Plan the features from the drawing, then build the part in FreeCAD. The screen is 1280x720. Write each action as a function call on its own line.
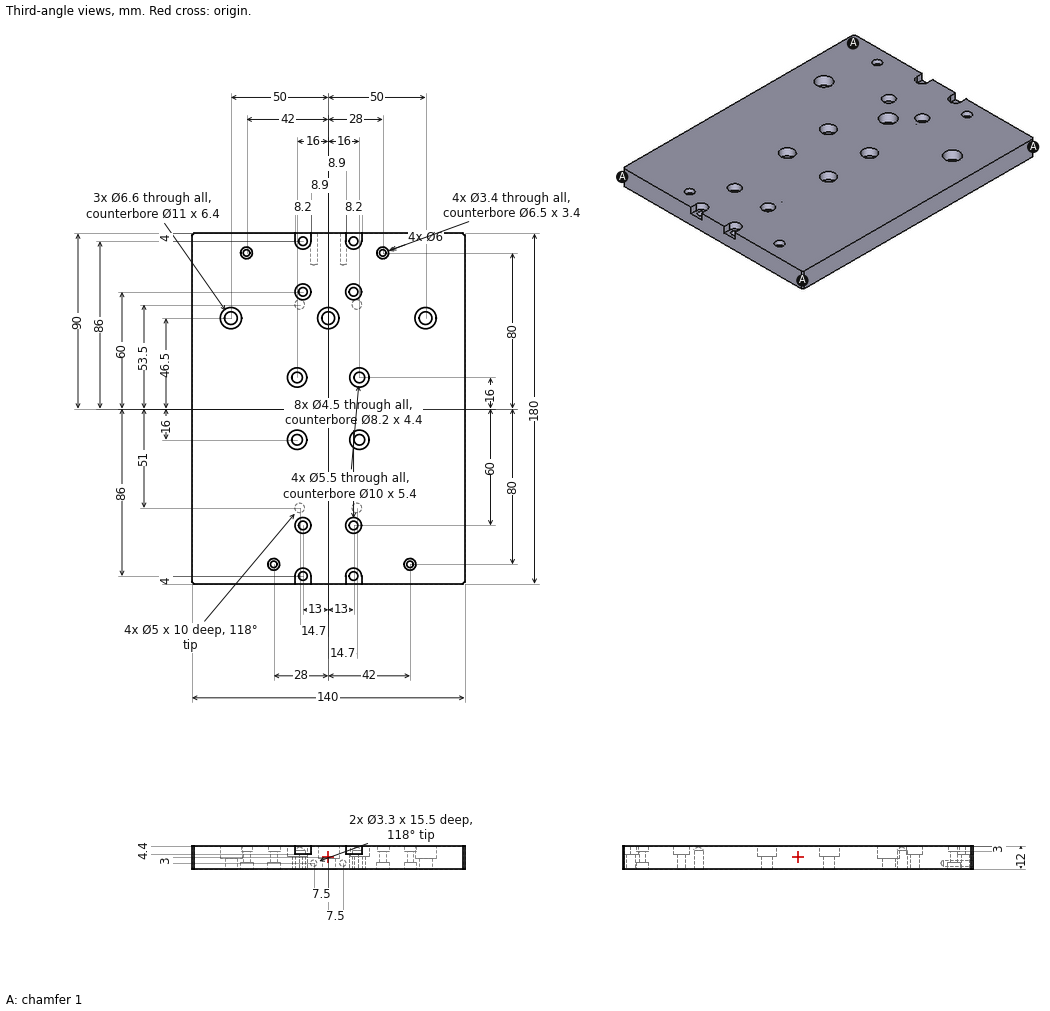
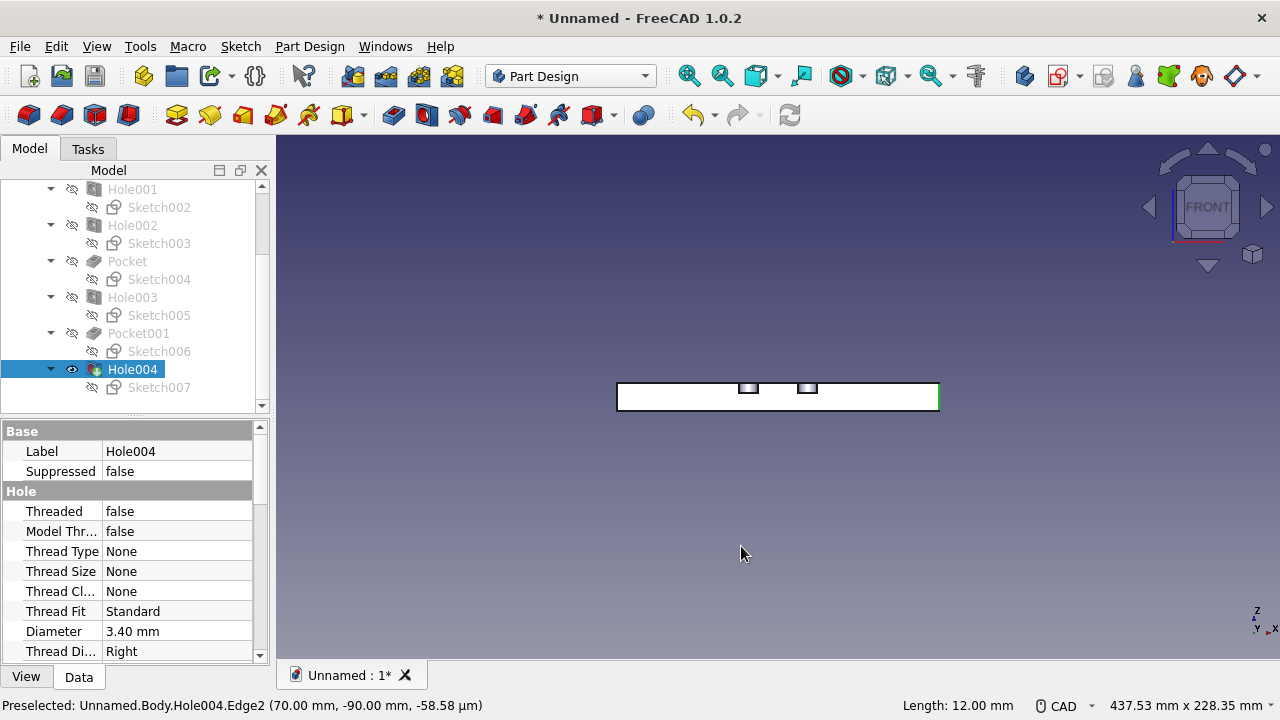
click(690, 76)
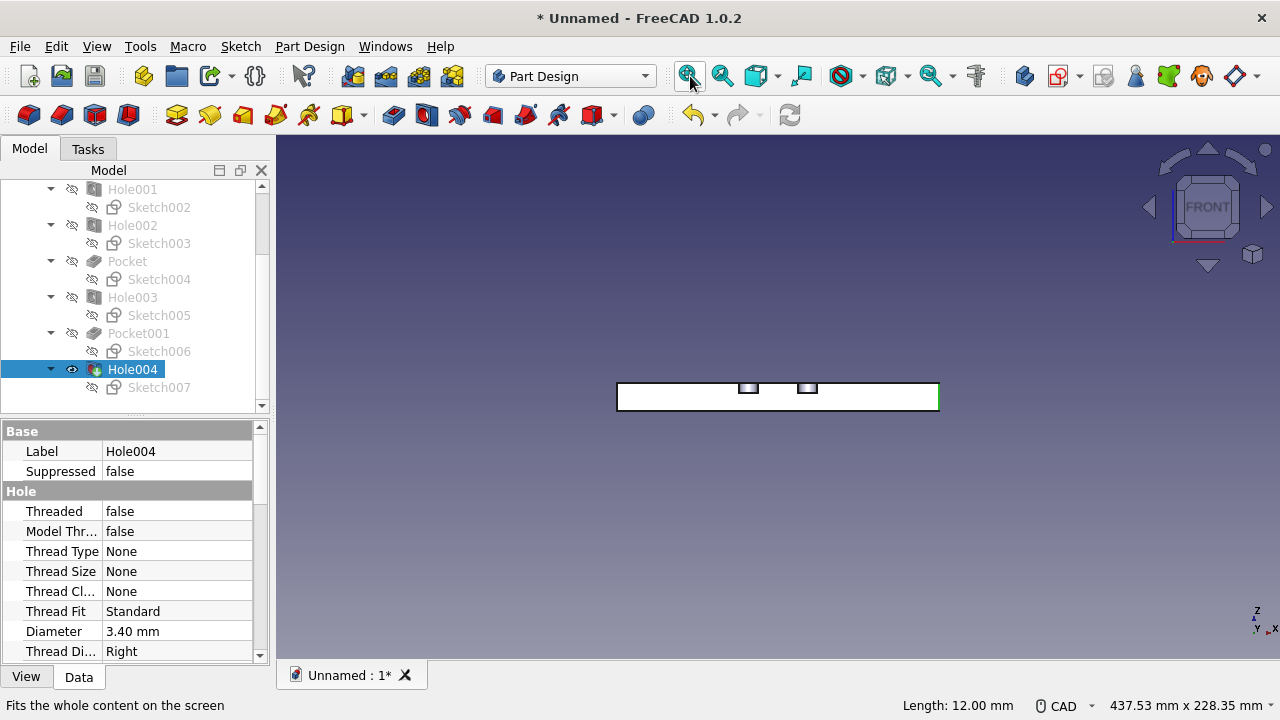
click(617, 396, ctrl)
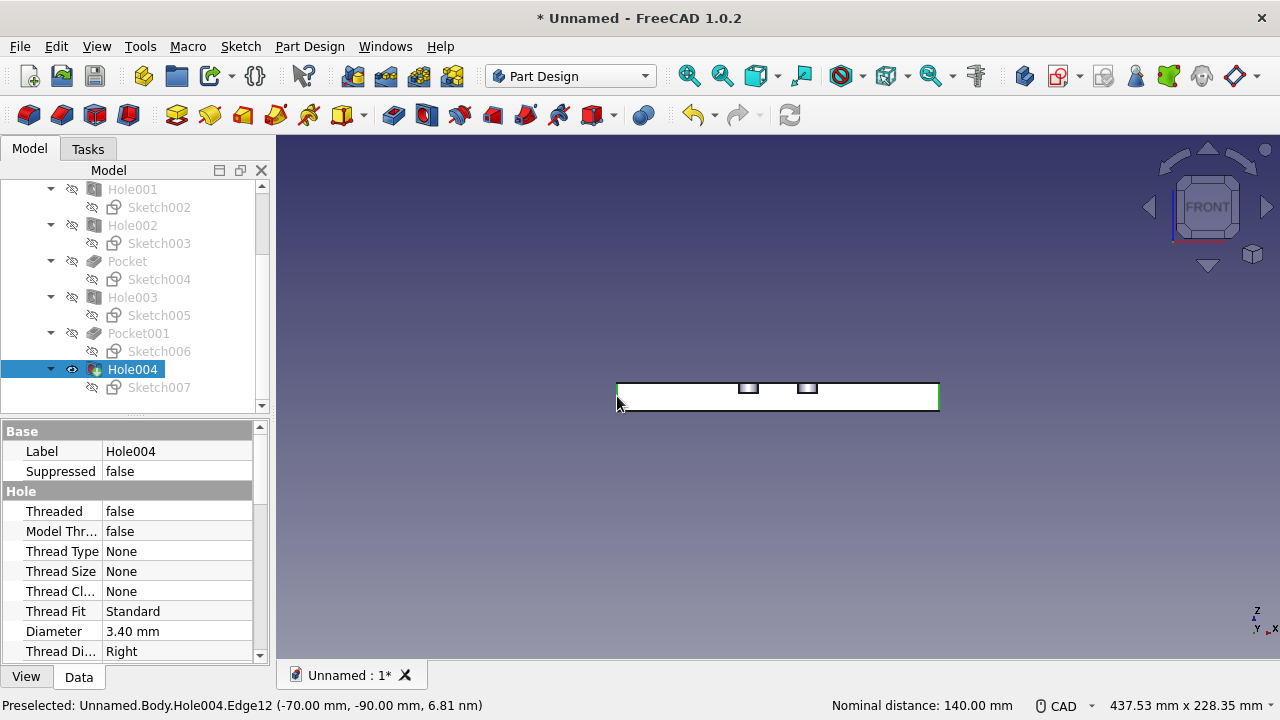
key(3)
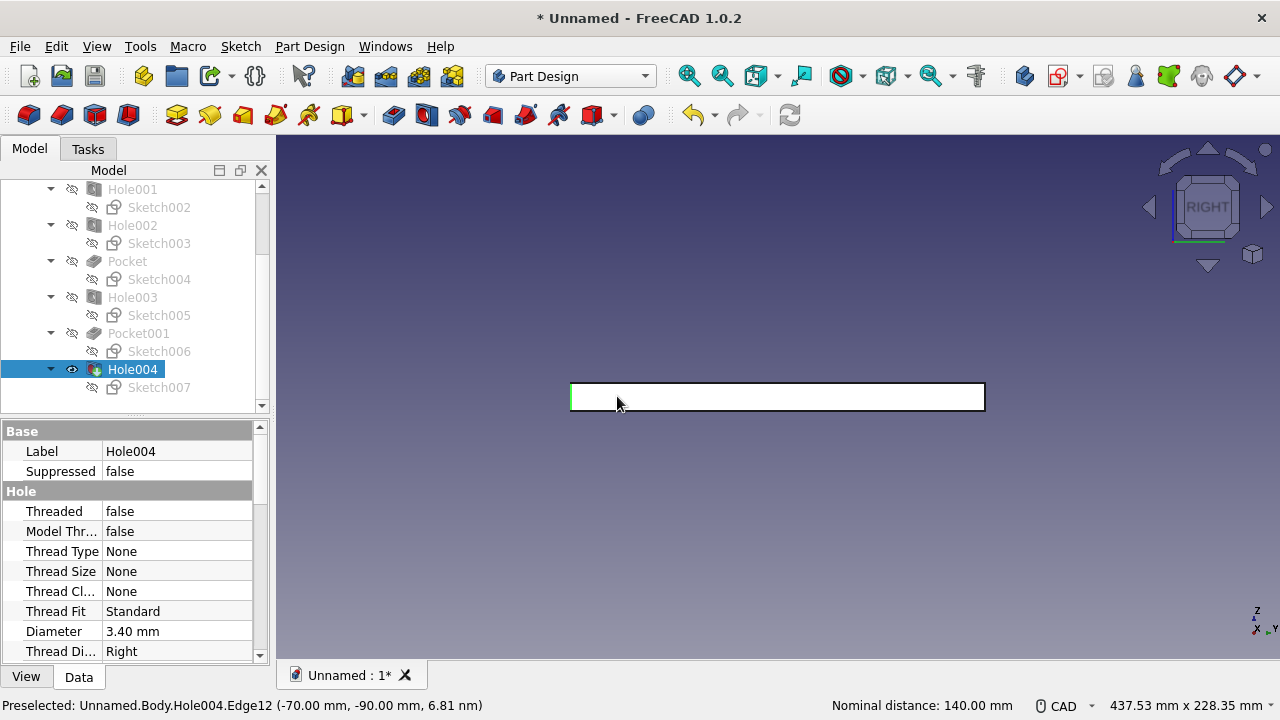
click(690, 76)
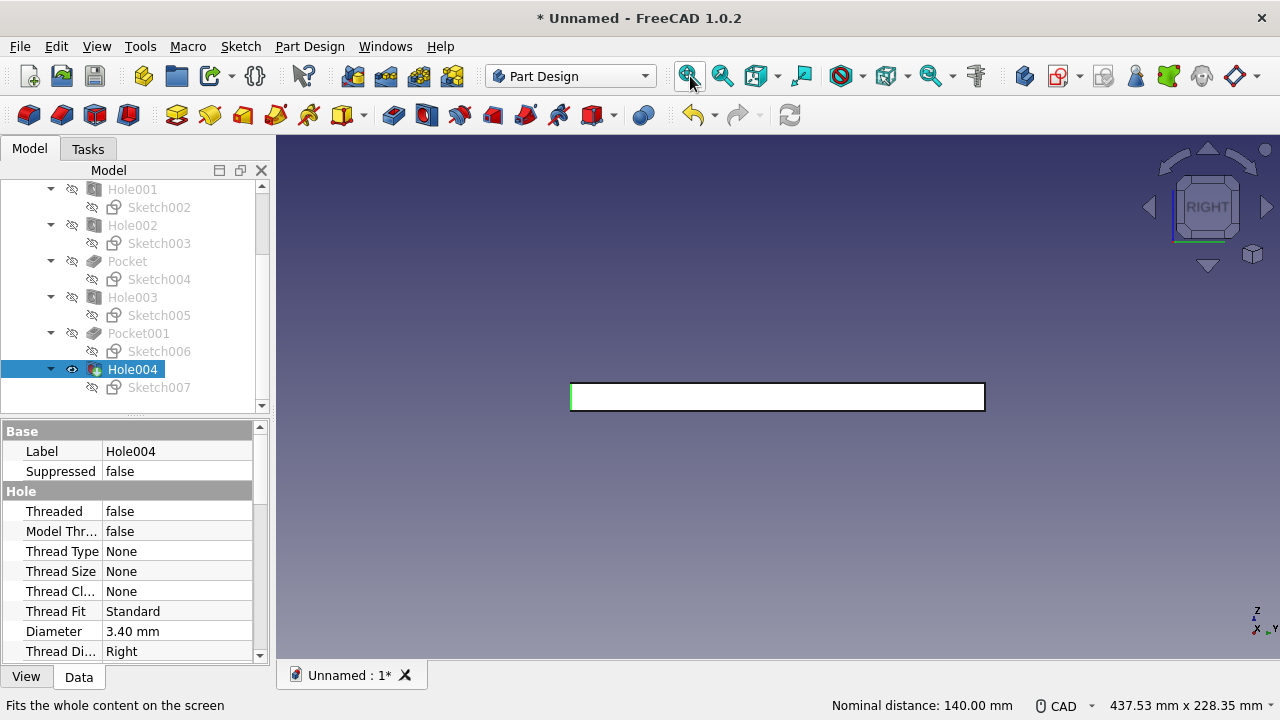
click(985, 396, ctrl)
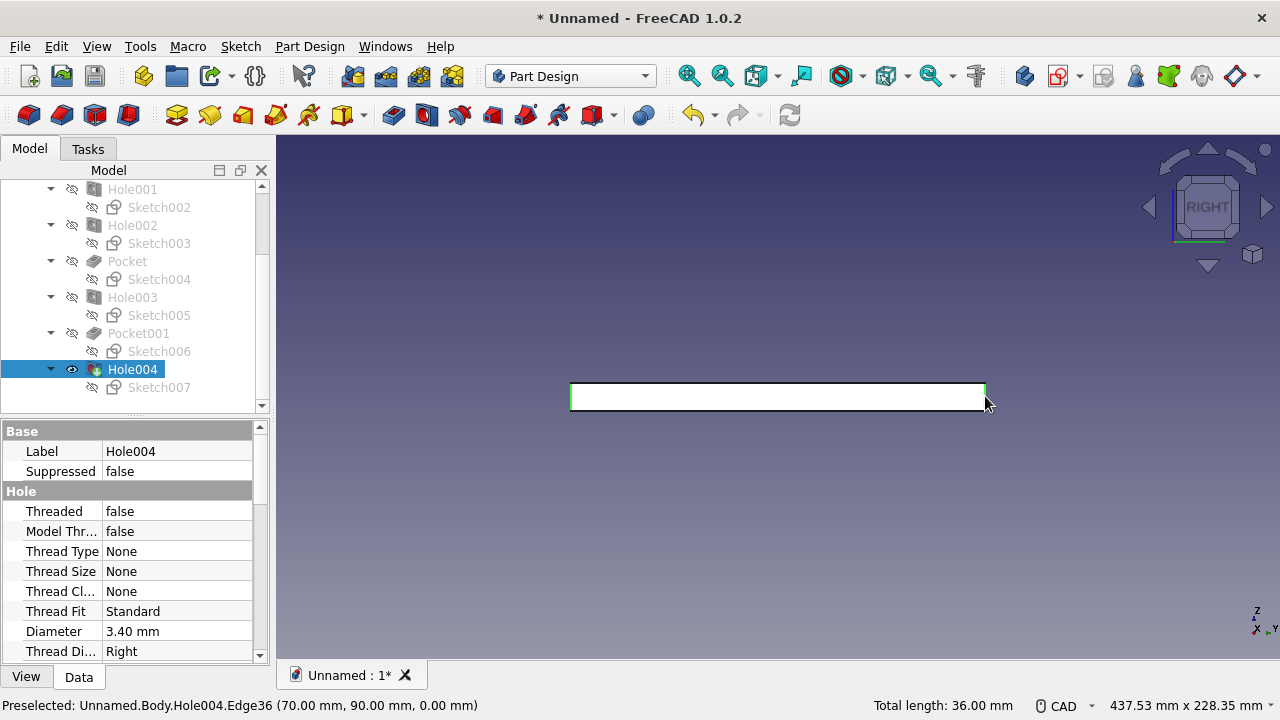
key(5)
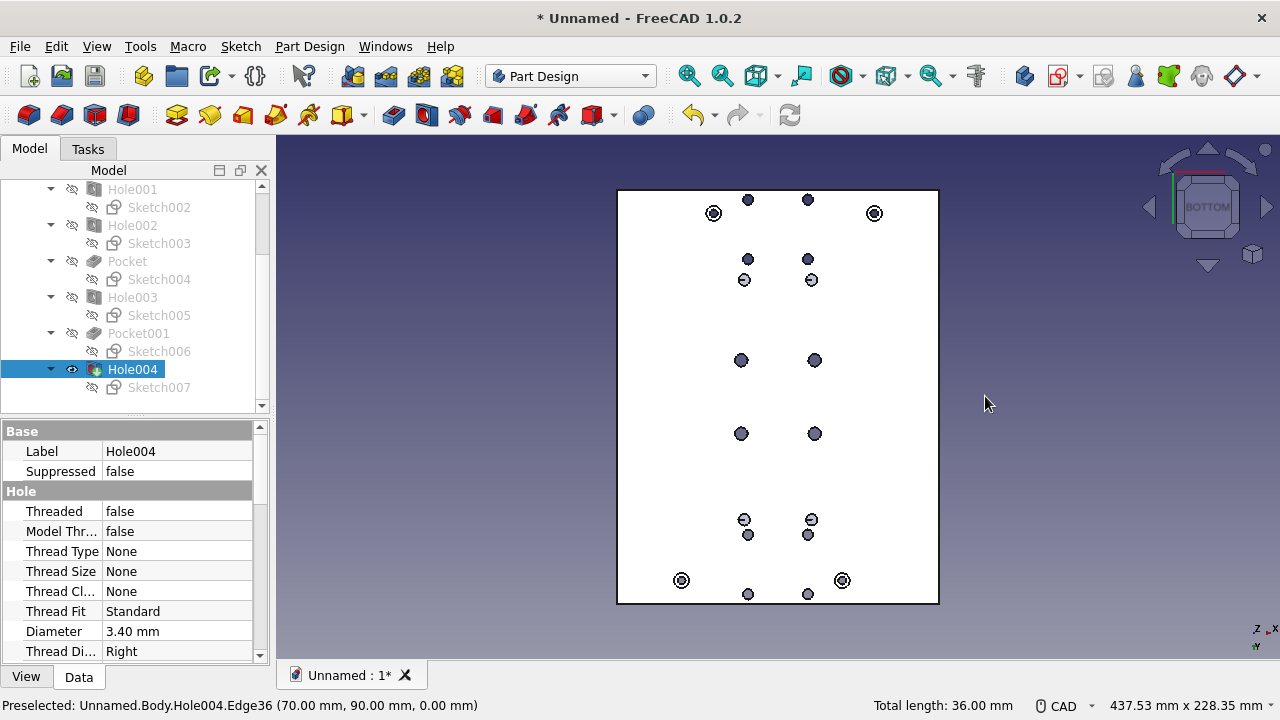
key(4)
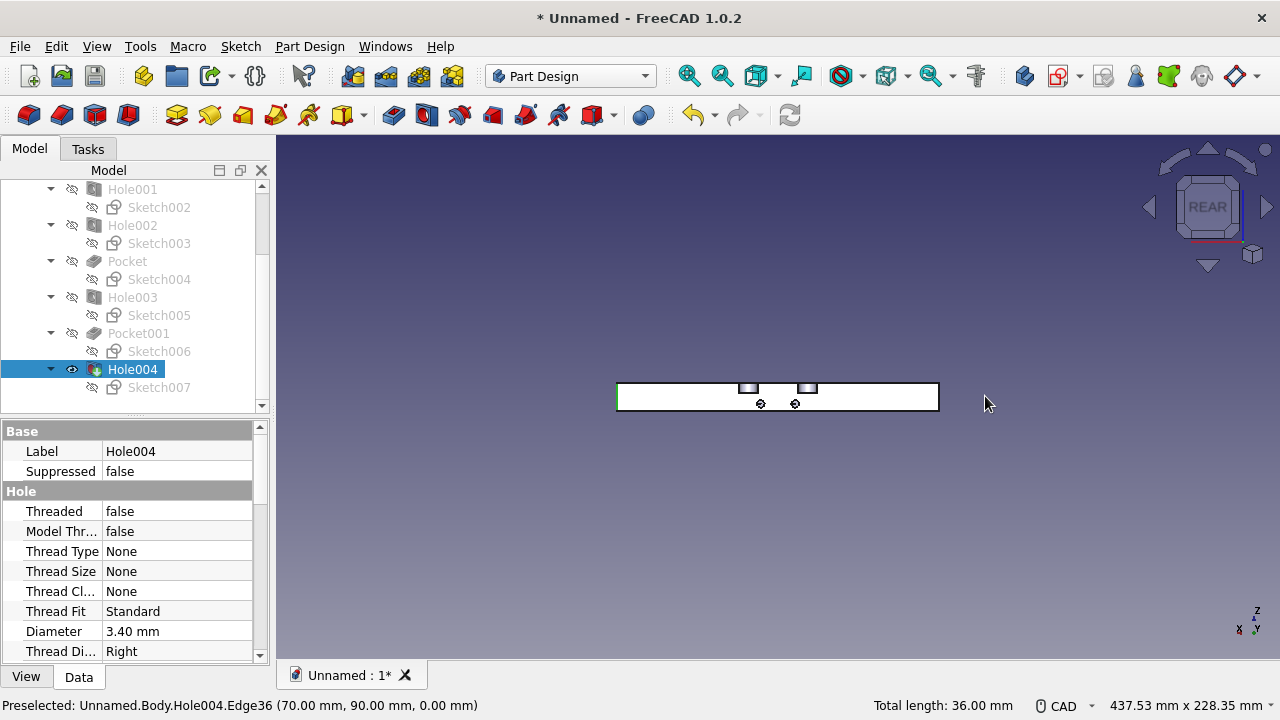
click(690, 76)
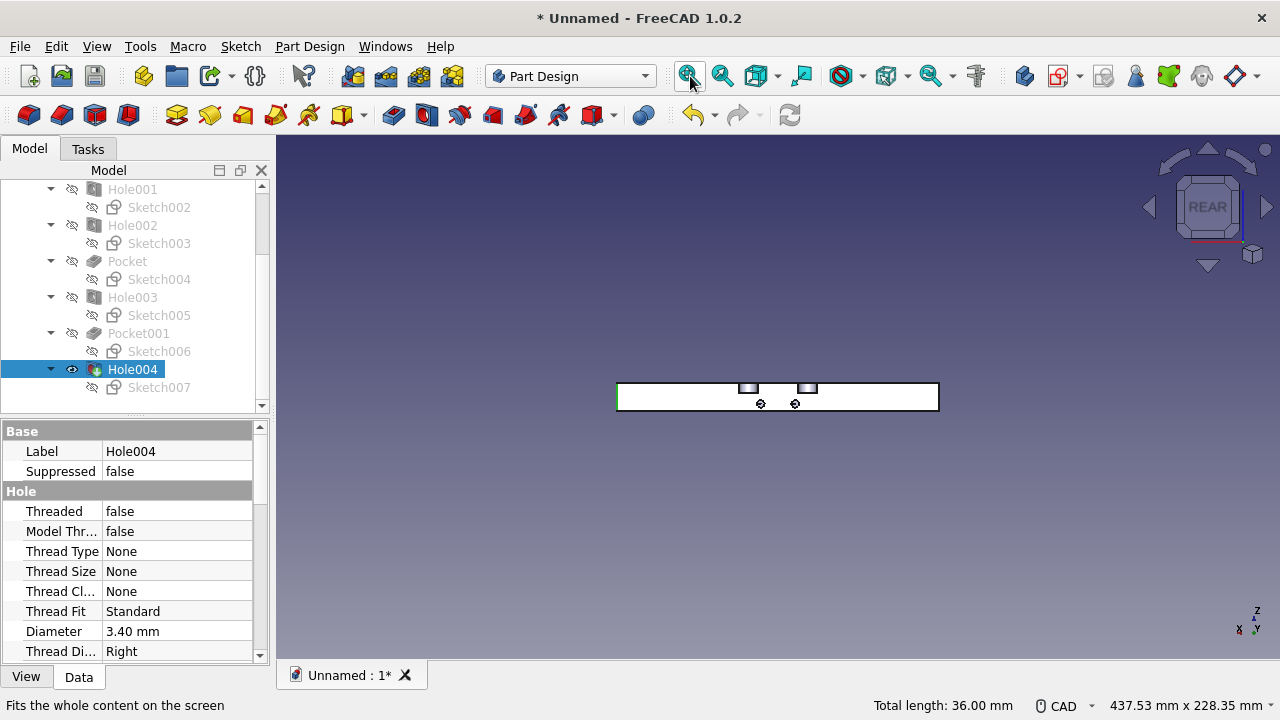
click(939, 396, ctrl)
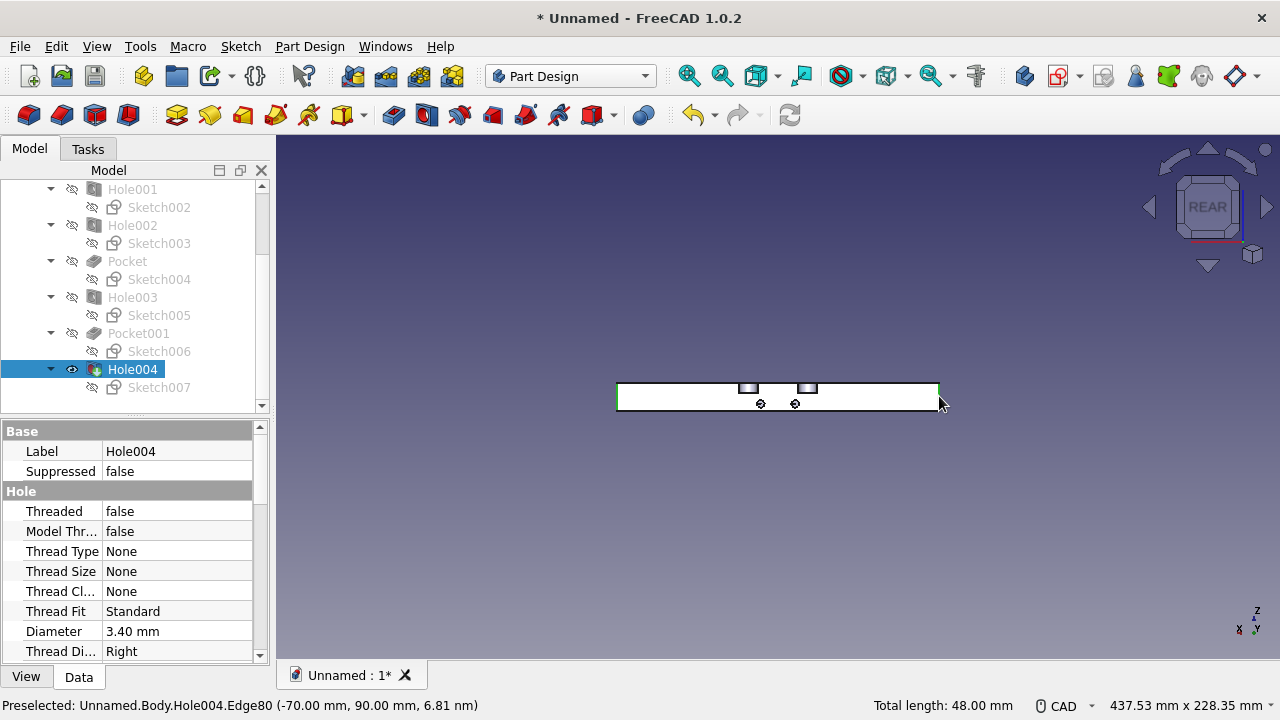
click(62, 116)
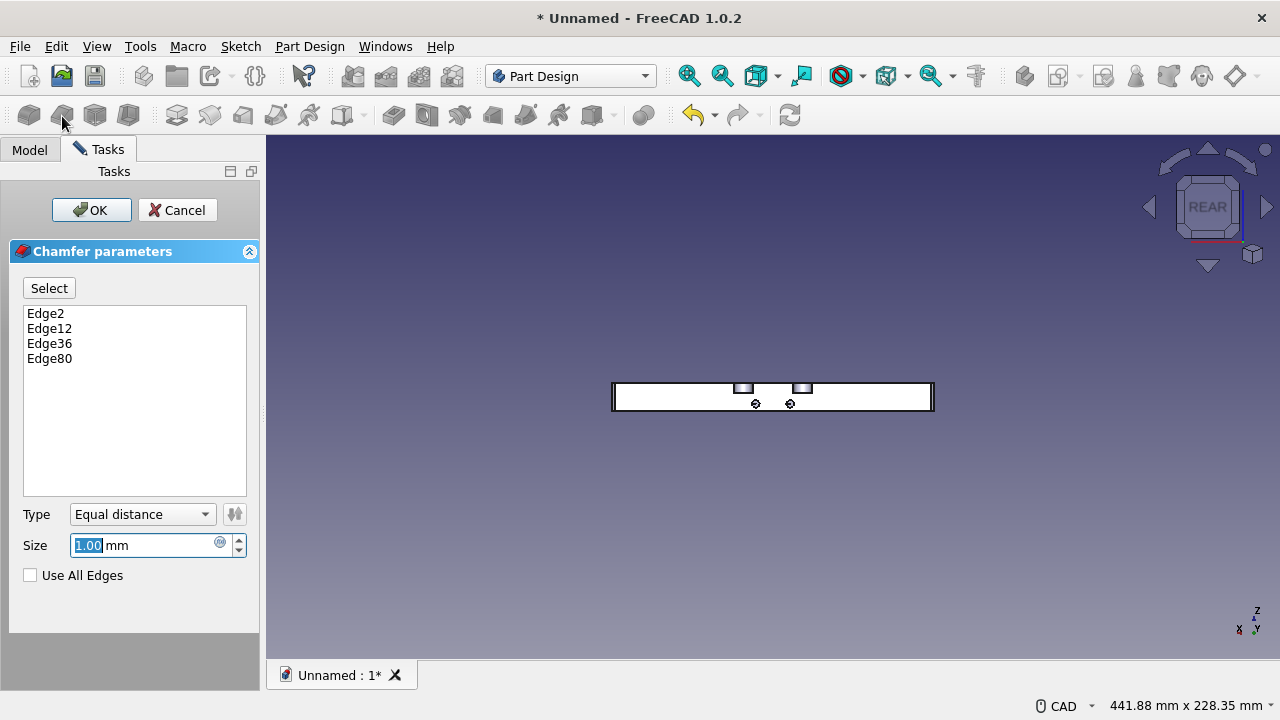
text(1)
key(Tab)